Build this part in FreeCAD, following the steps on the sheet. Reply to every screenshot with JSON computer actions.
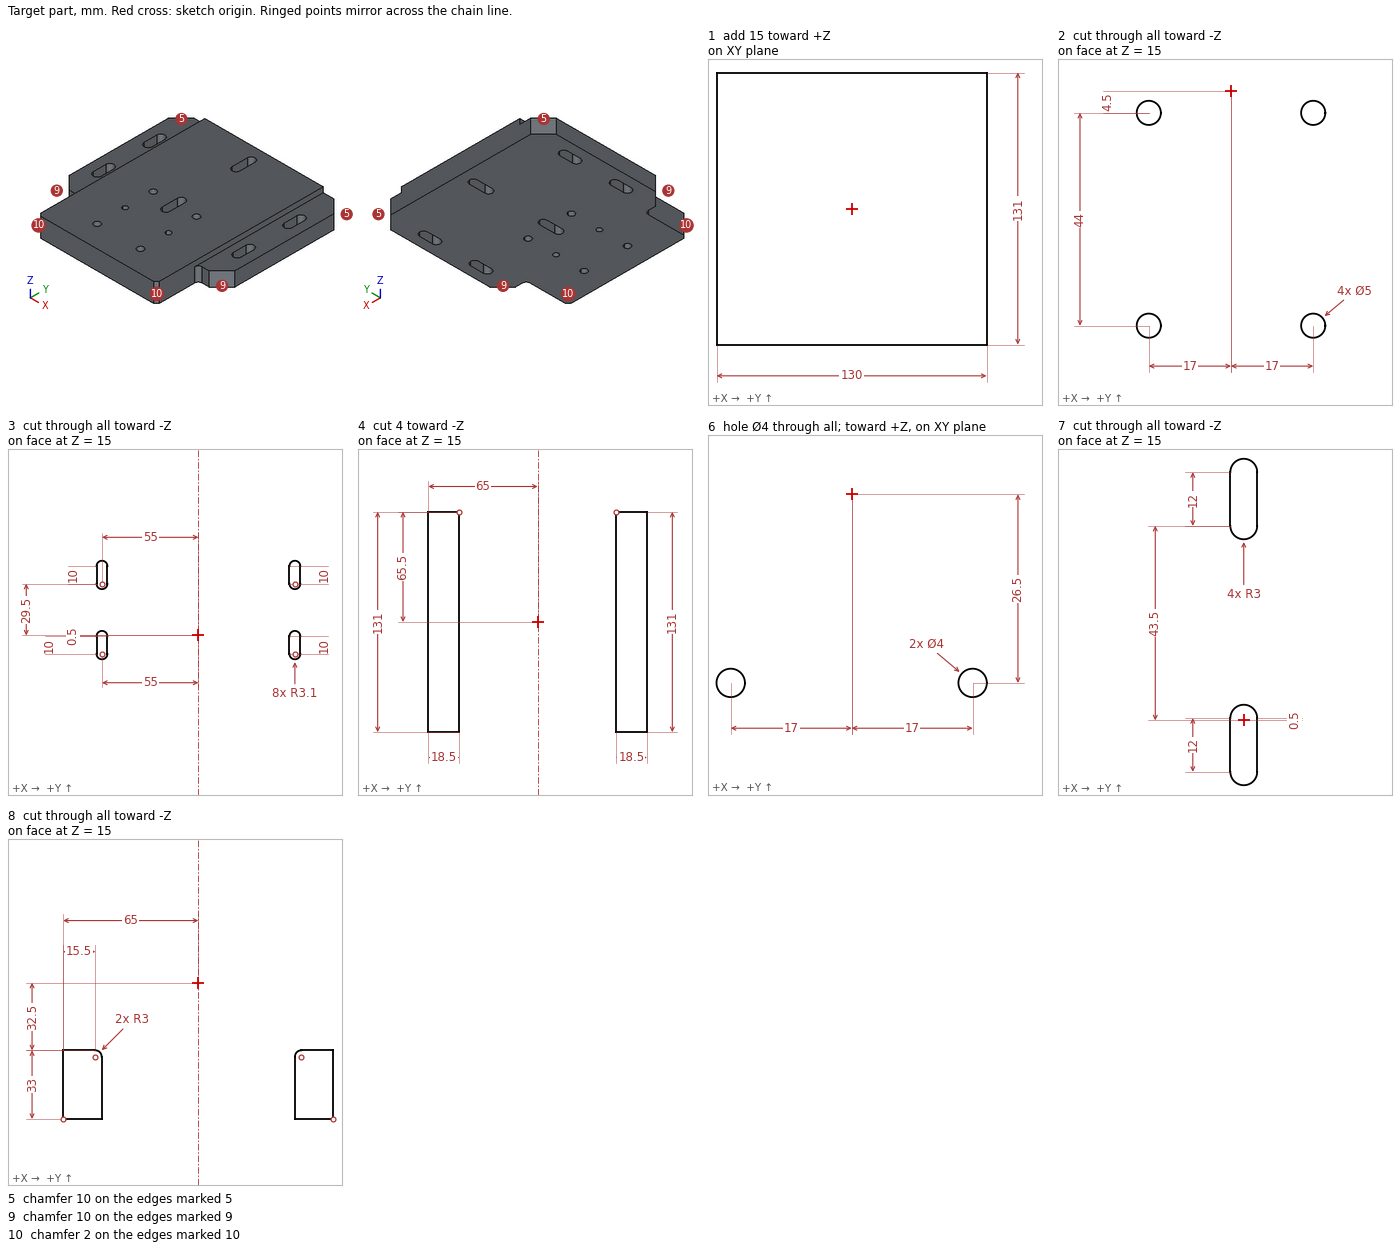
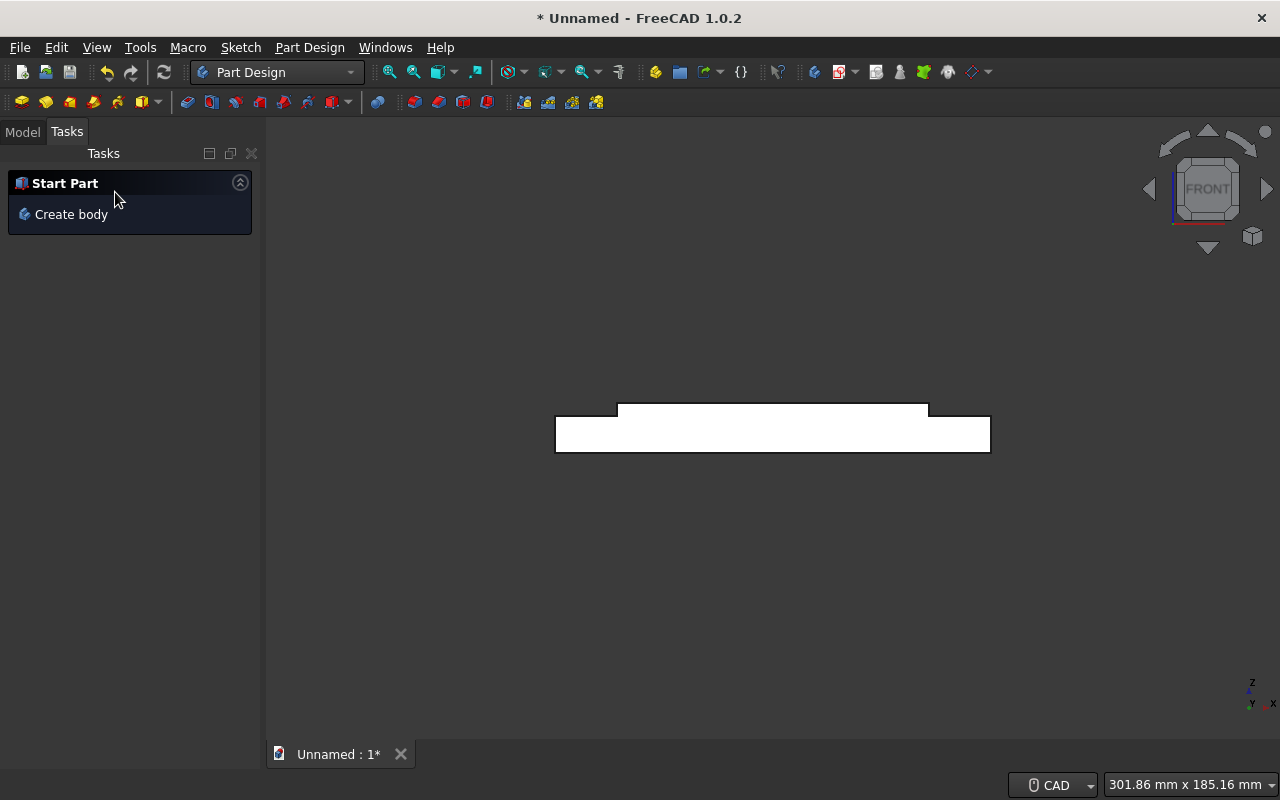
{"action": "key", "text": "3"}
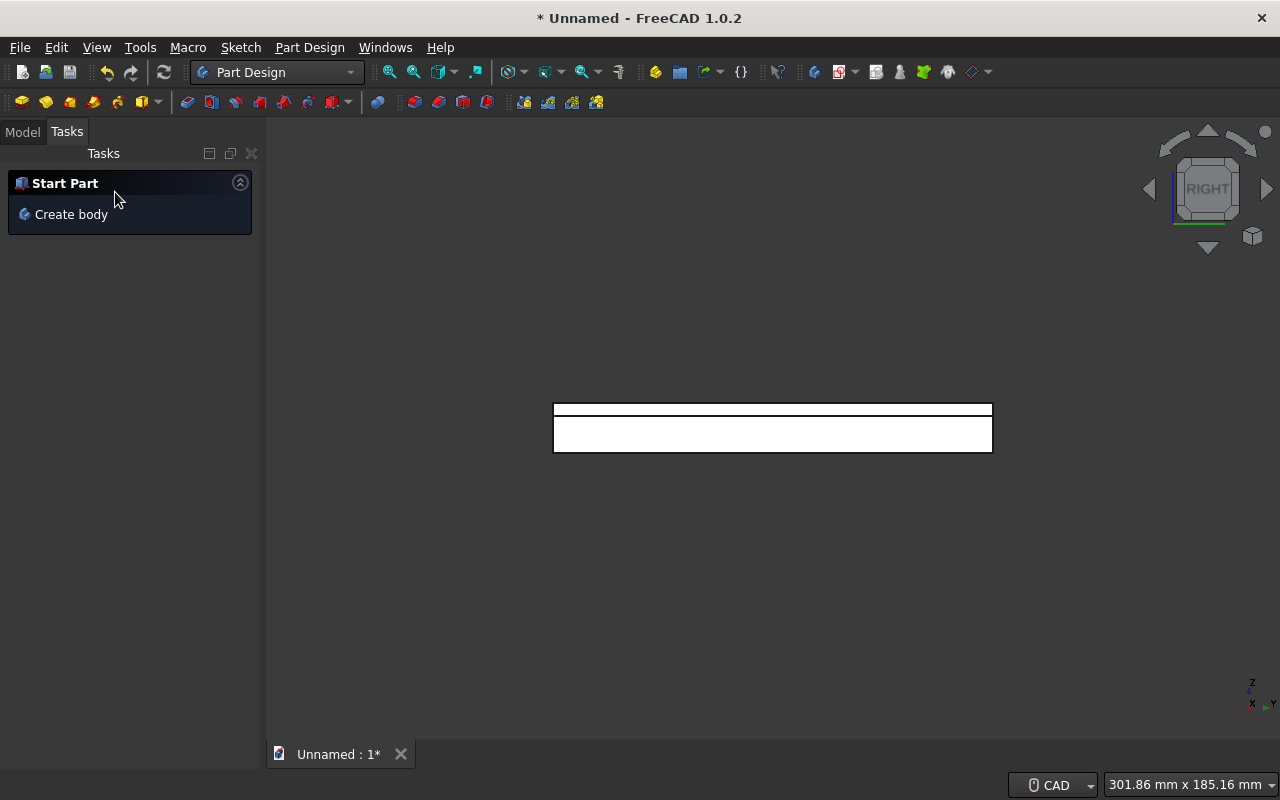
{"action": "key", "text": "v f"}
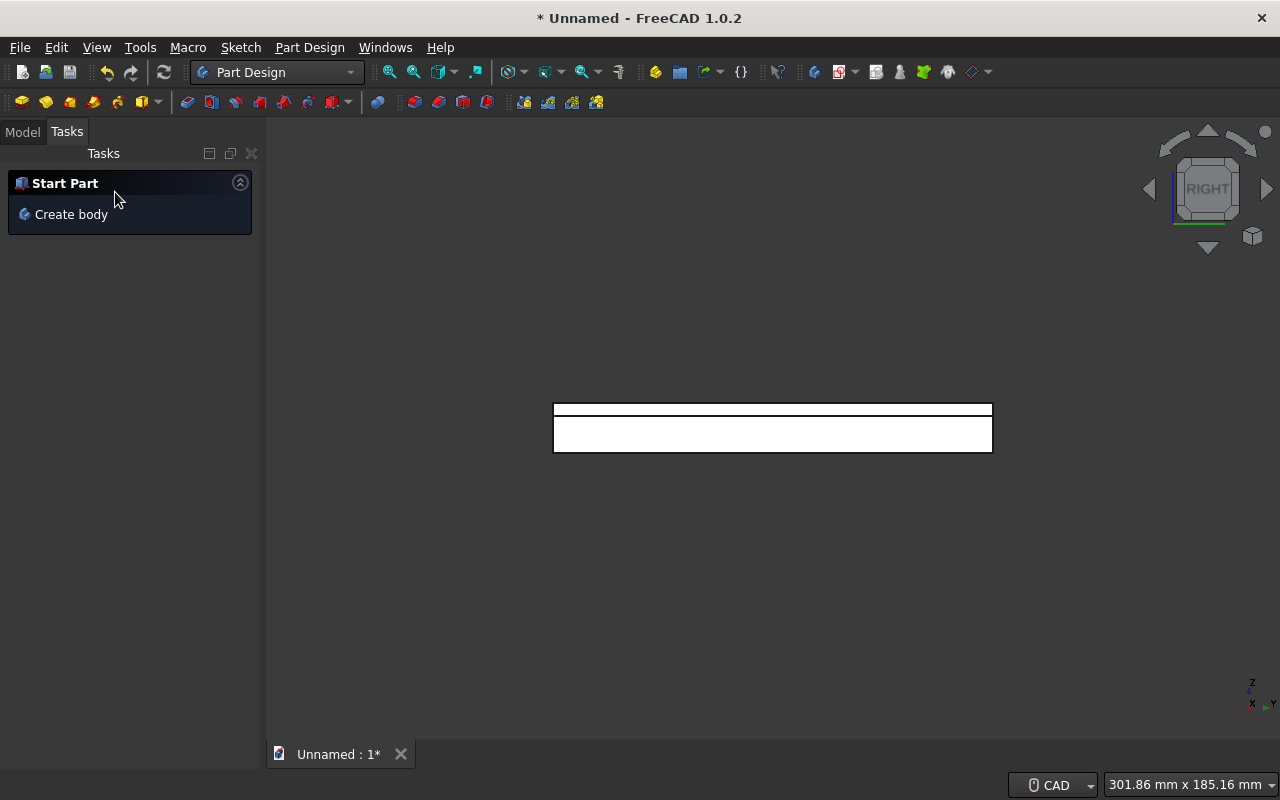
{"action": "left_click", "coordinate": [993, 434]}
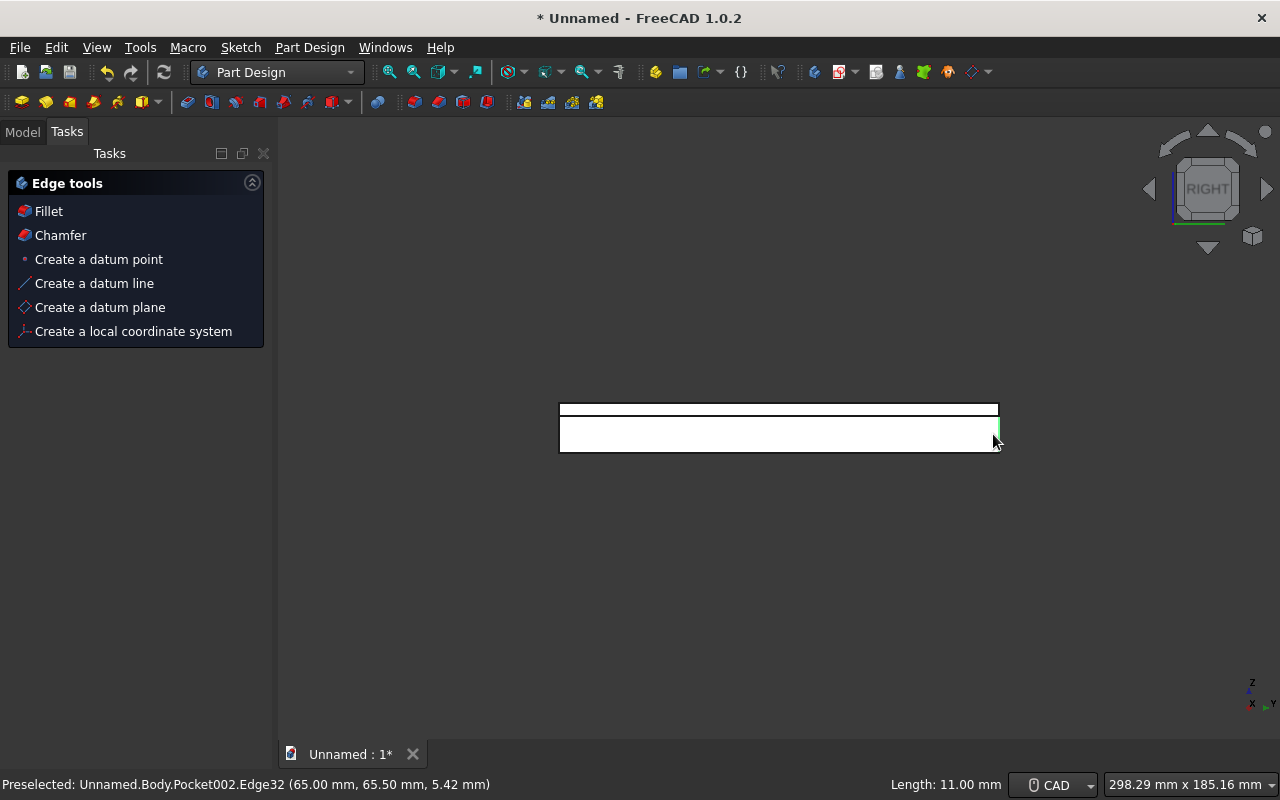
{"action": "key", "text": "5"}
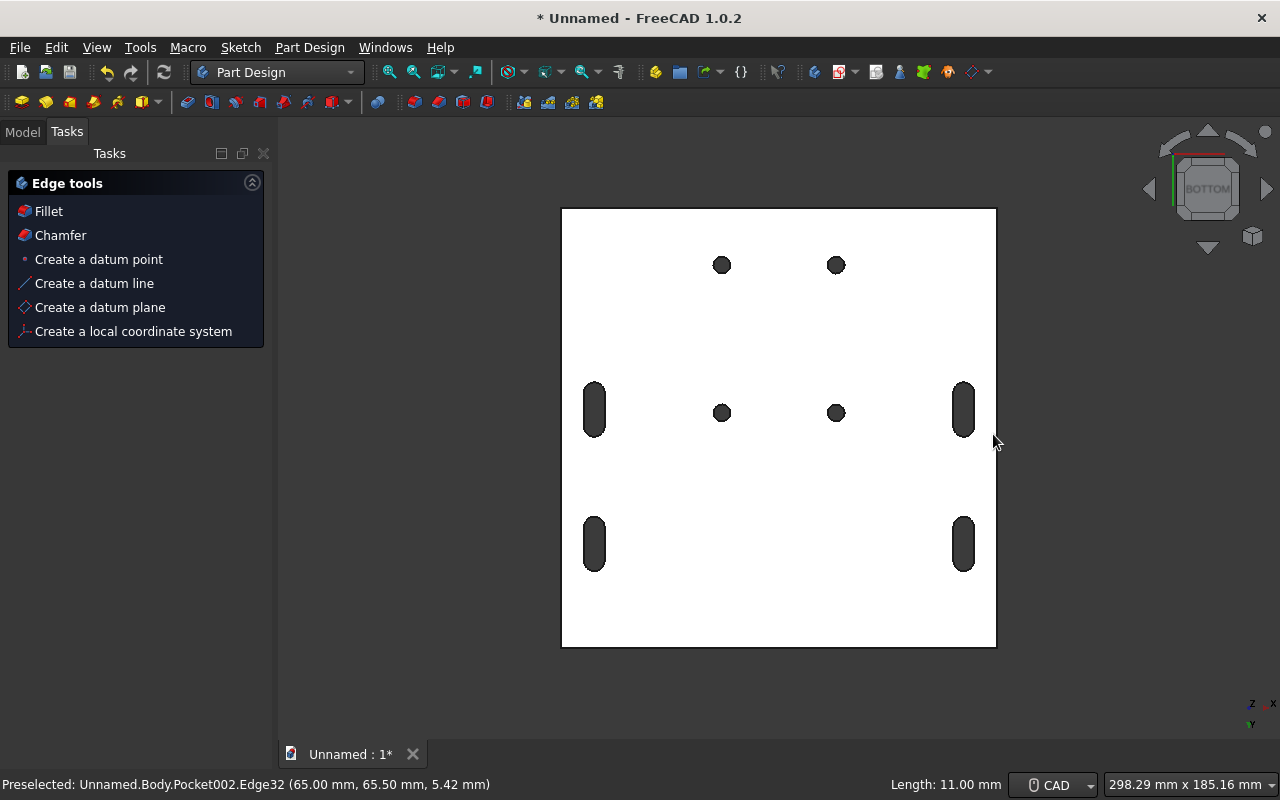
{"action": "key", "text": "4"}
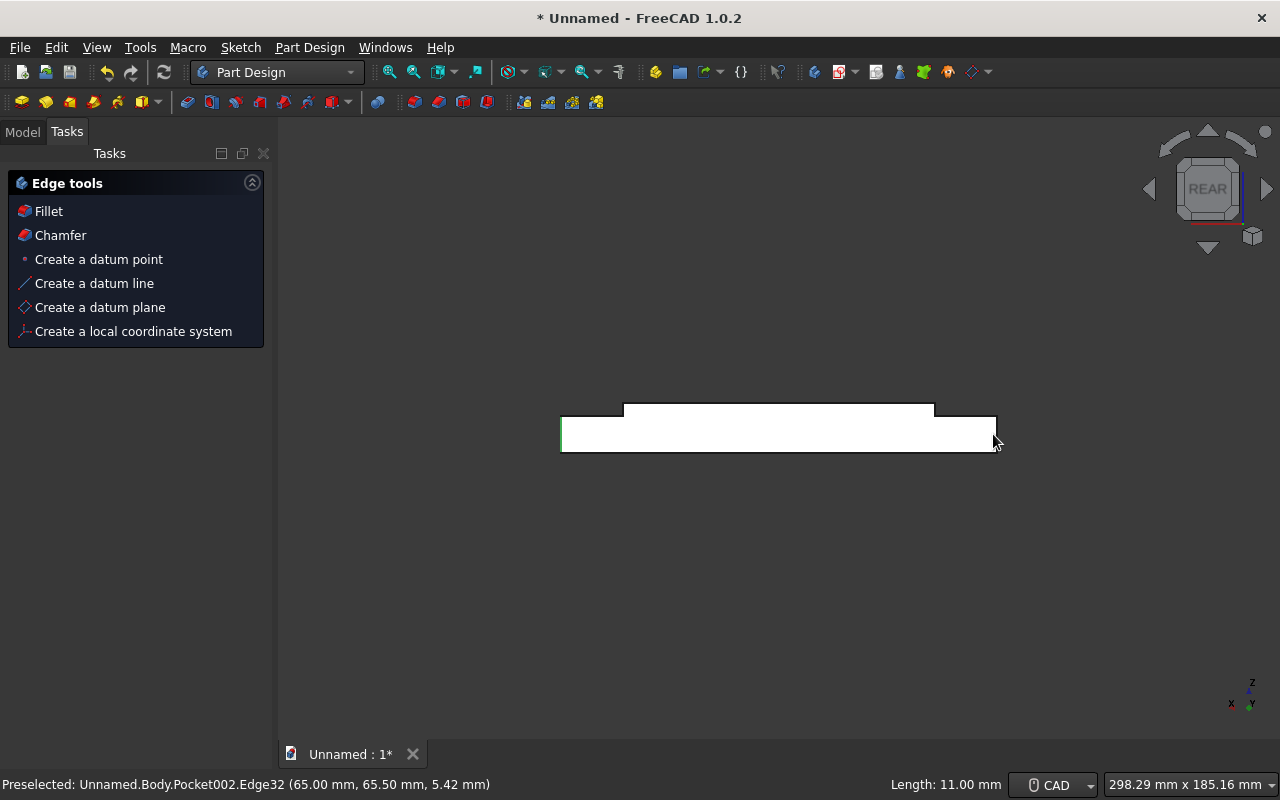
{"action": "key", "text": "v f"}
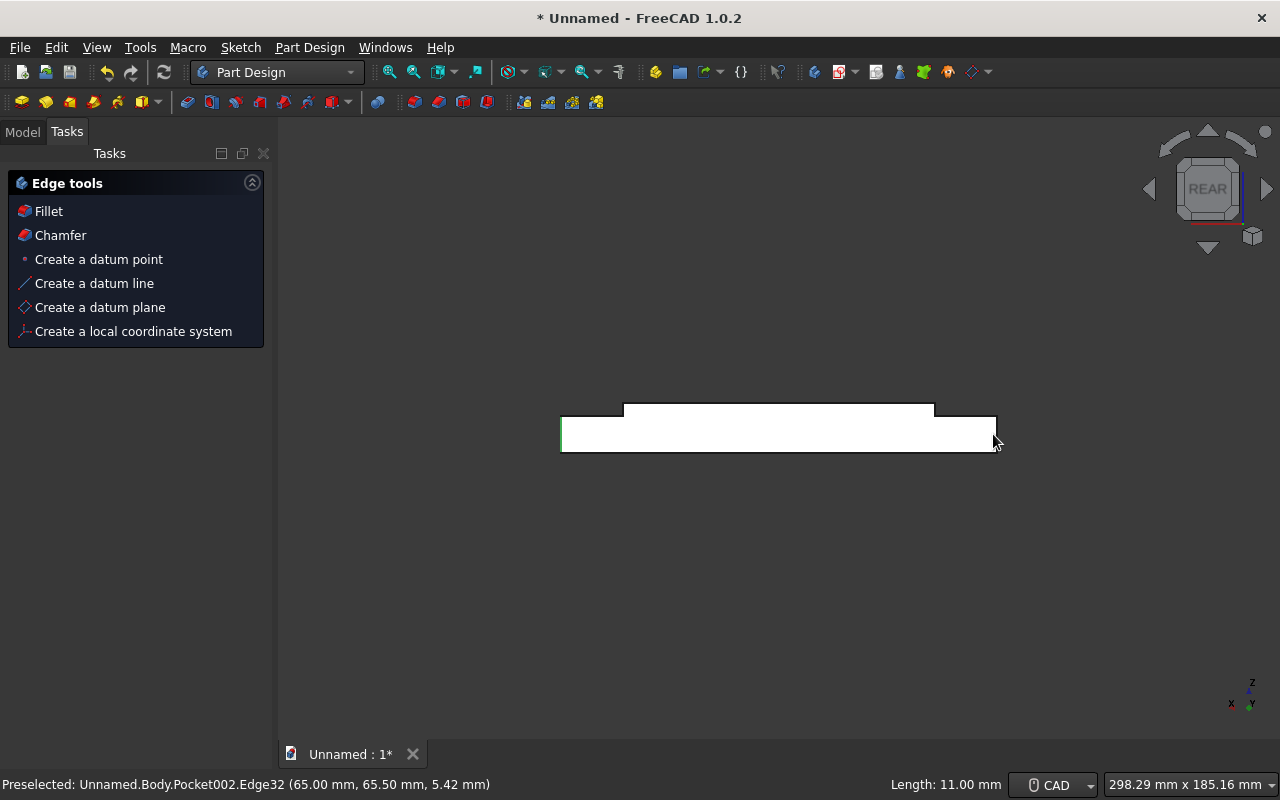
{"action": "left_click", "coordinate": [997, 434], "text": "ctrl"}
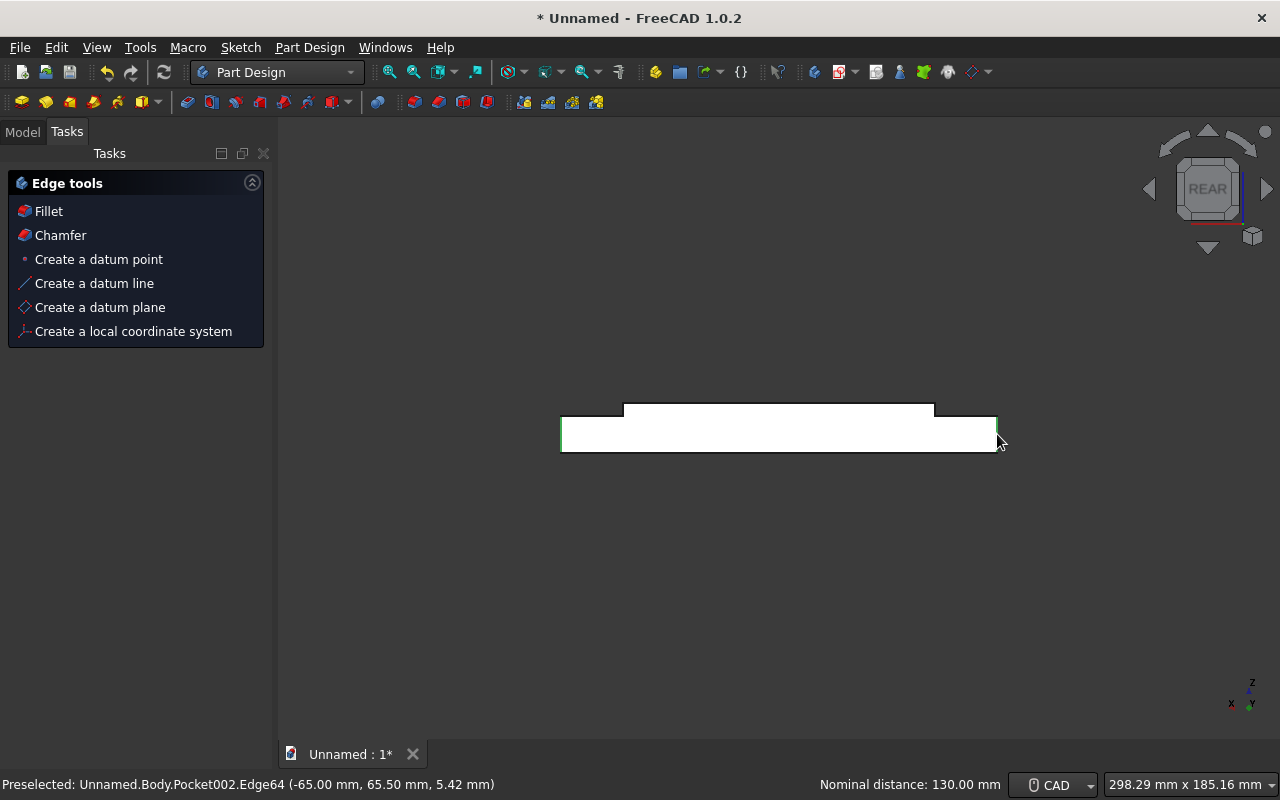
{"action": "left_click", "coordinate": [440, 102]}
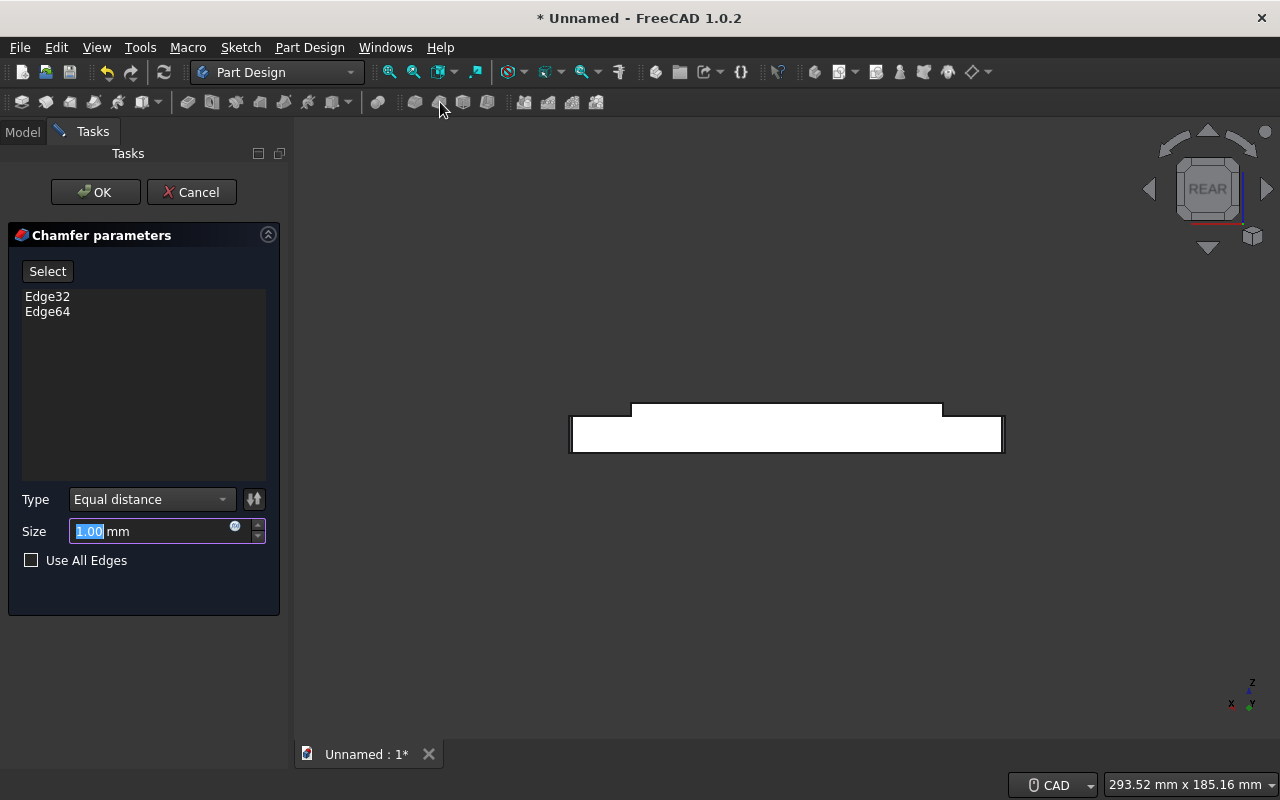
{"action": "type", "text": "10"}
{"action": "key", "text": "Tab"}